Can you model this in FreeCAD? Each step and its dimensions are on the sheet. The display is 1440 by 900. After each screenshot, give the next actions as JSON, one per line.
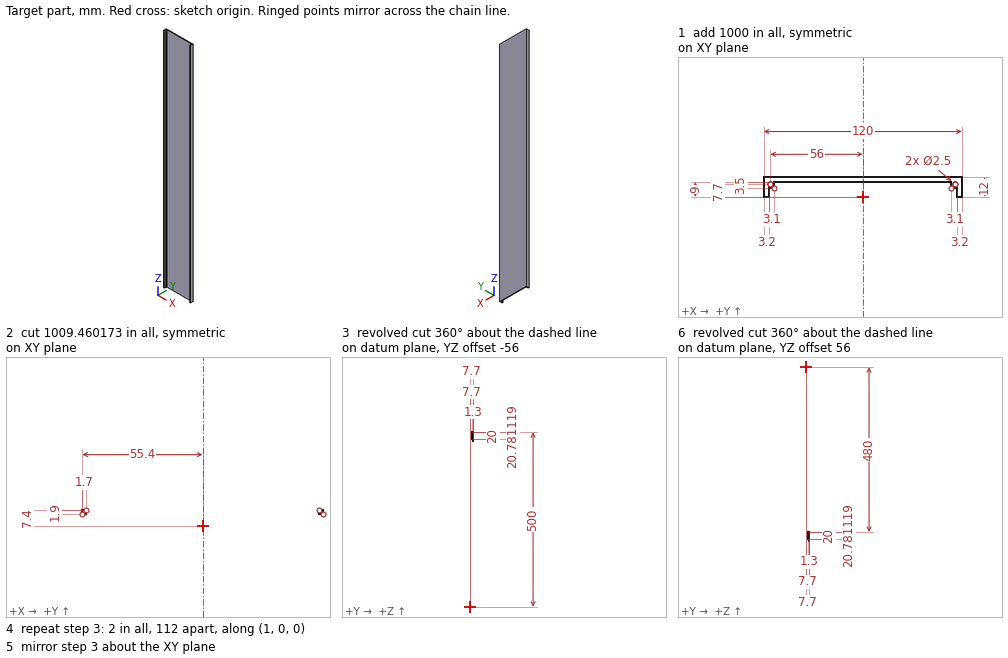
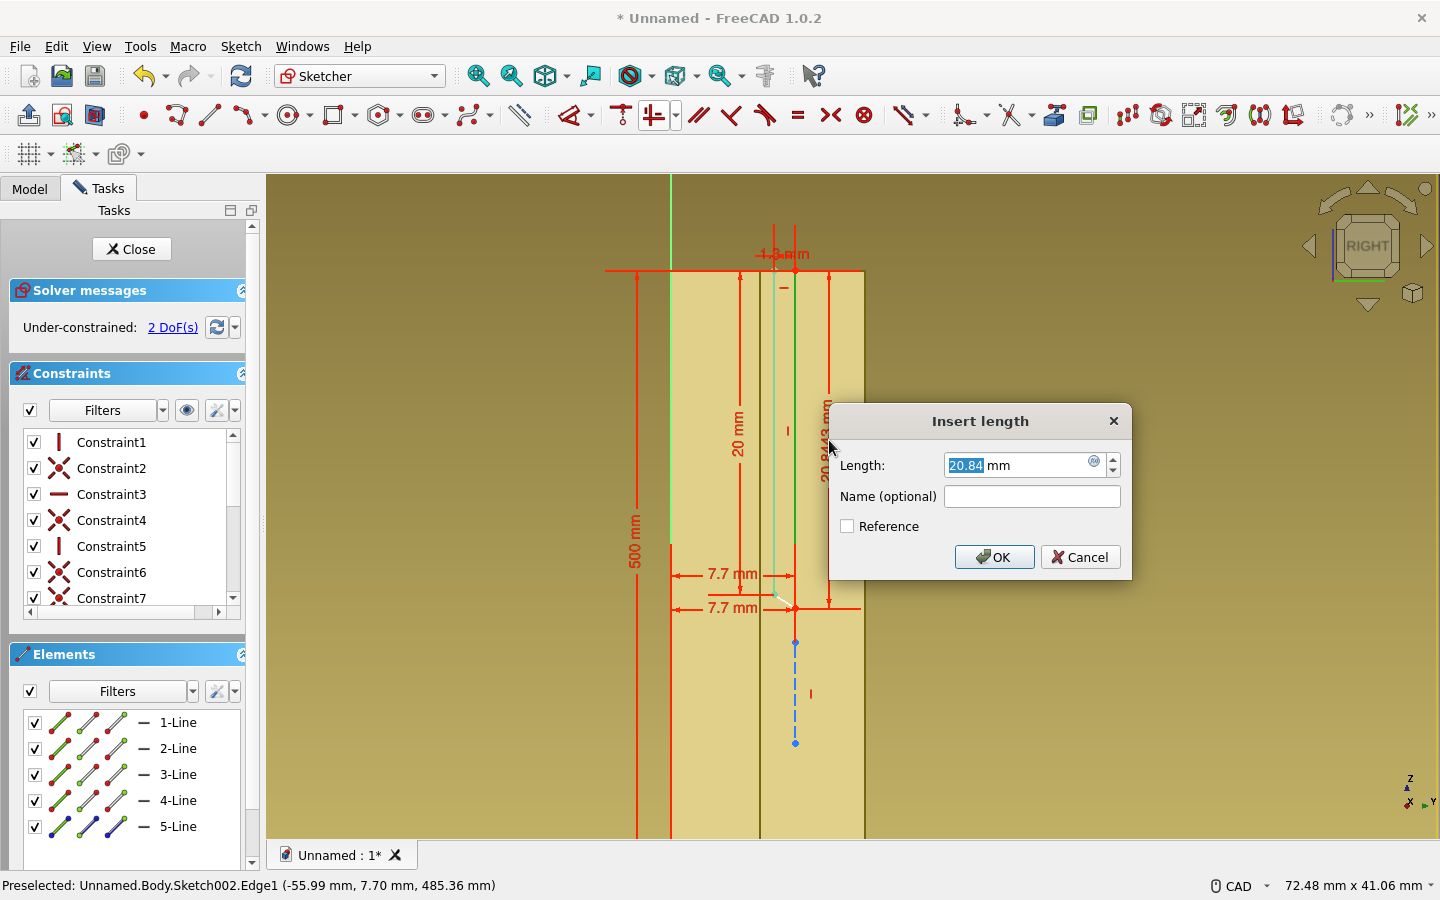
{"action": "type", "text": "20.781119"}
{"action": "key", "text": "Return"}
{"action": "key", "text": "Escape"}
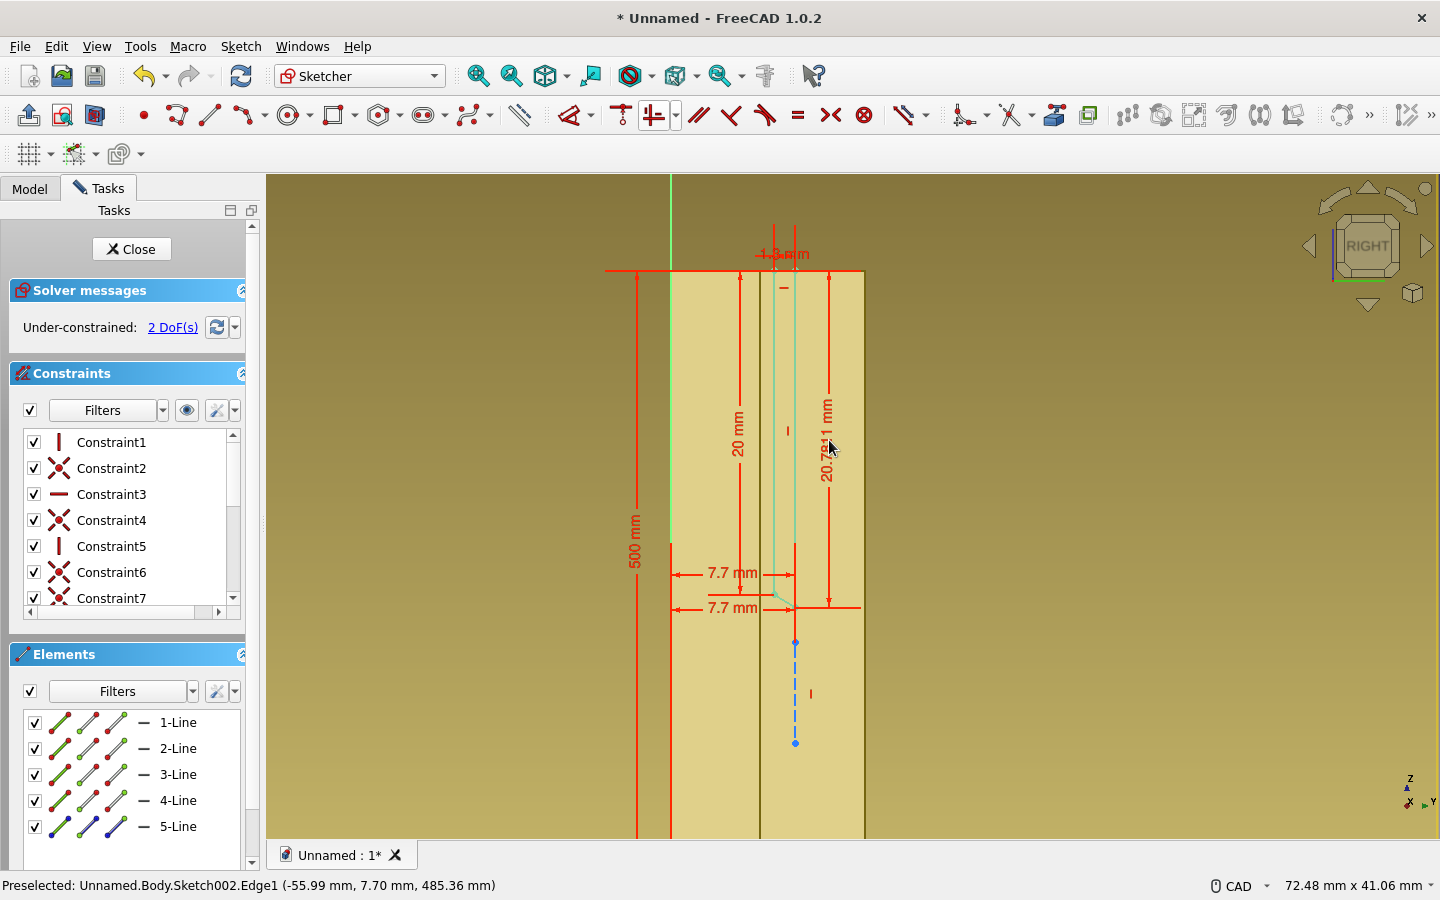
{"action": "left_click", "coordinate": [132, 249]}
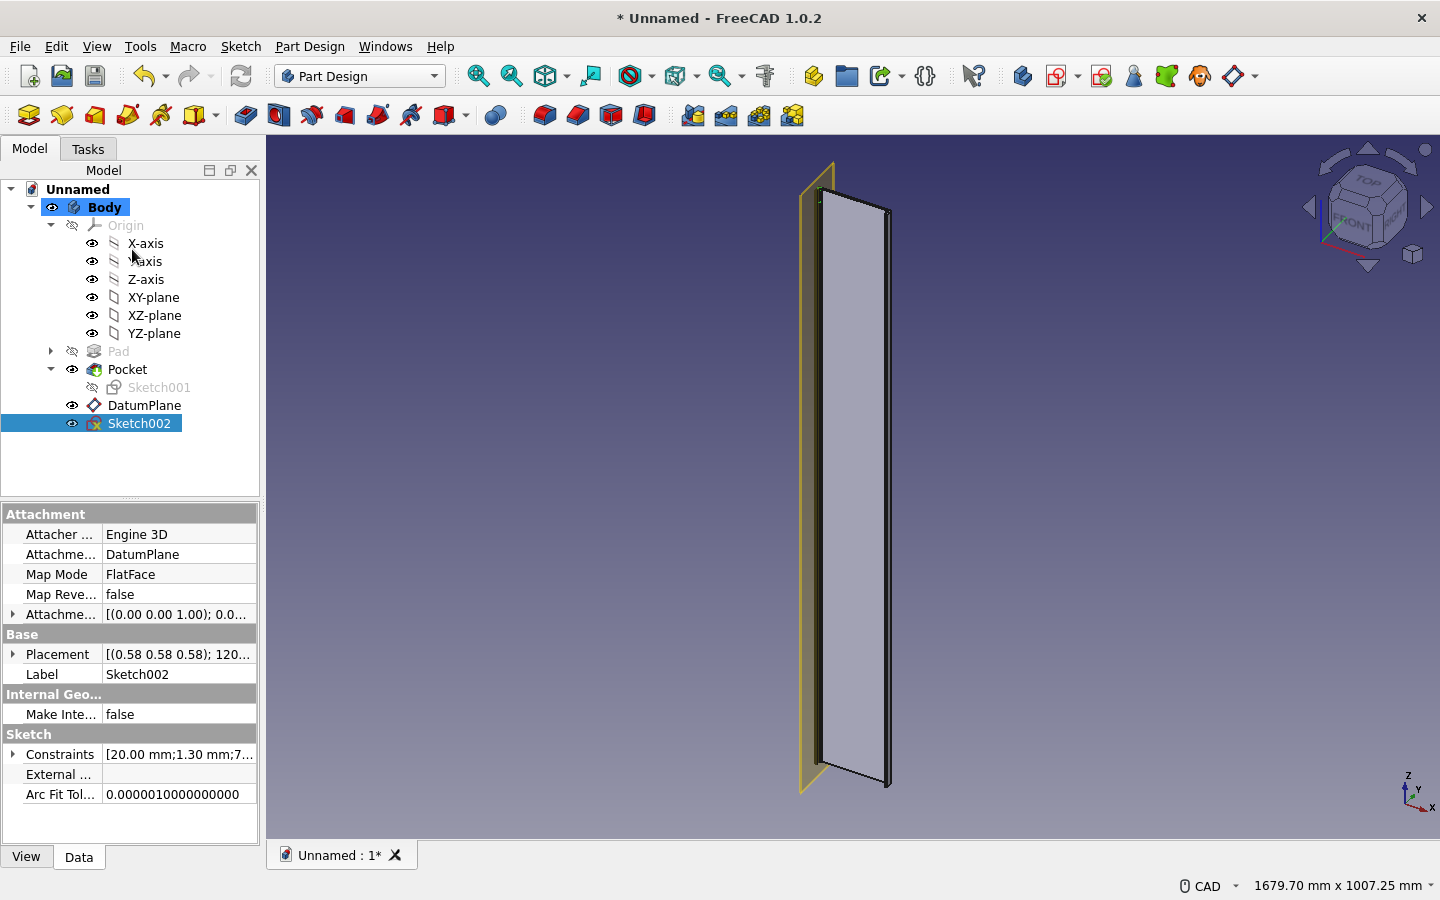
{"action": "left_click", "coordinate": [312, 116]}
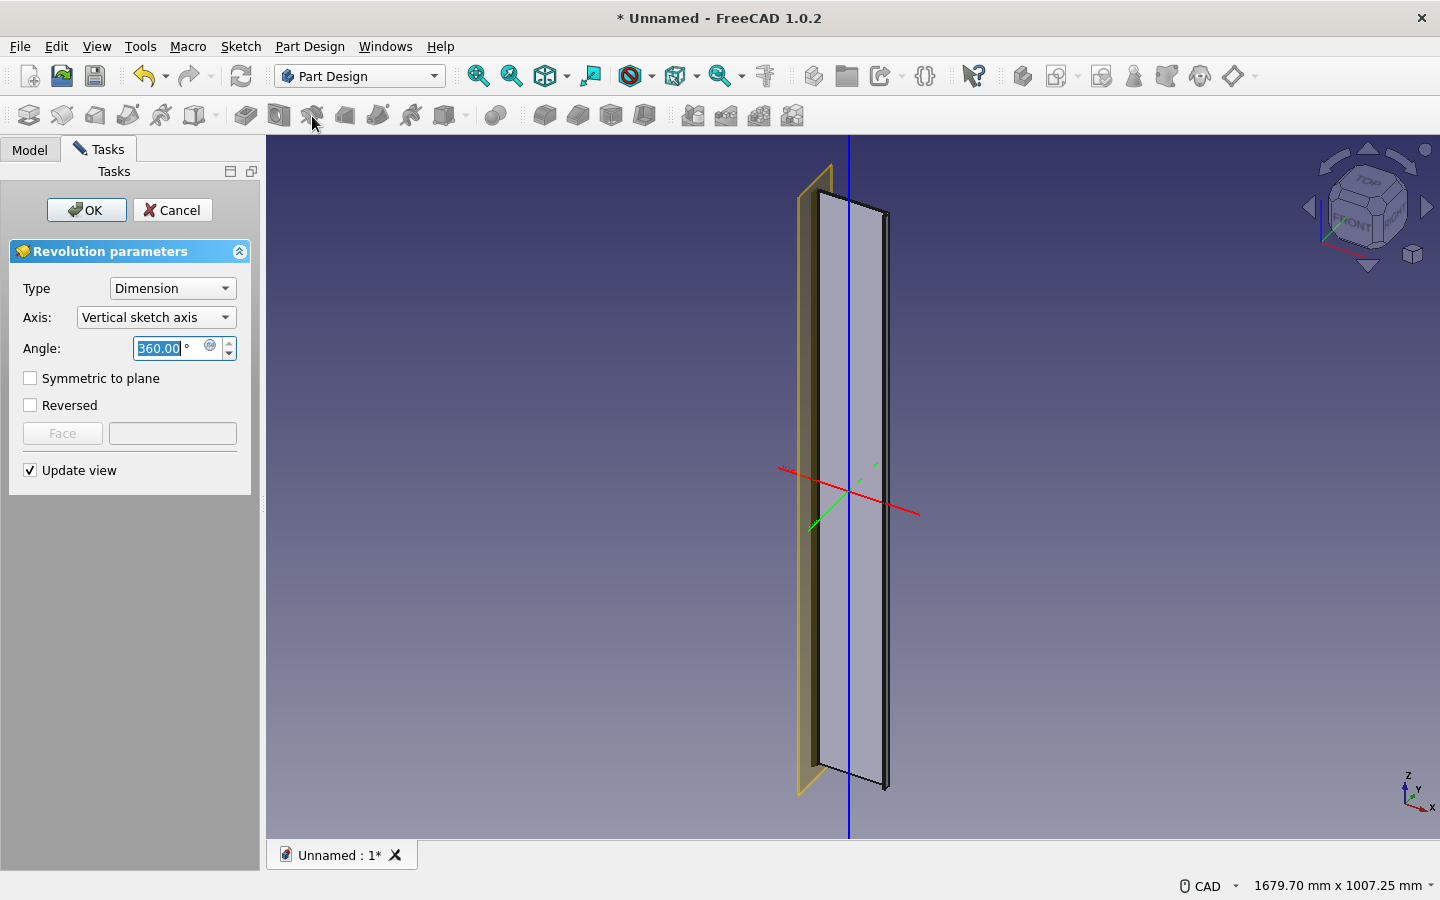
{"action": "left_click", "coordinate": [157, 318]}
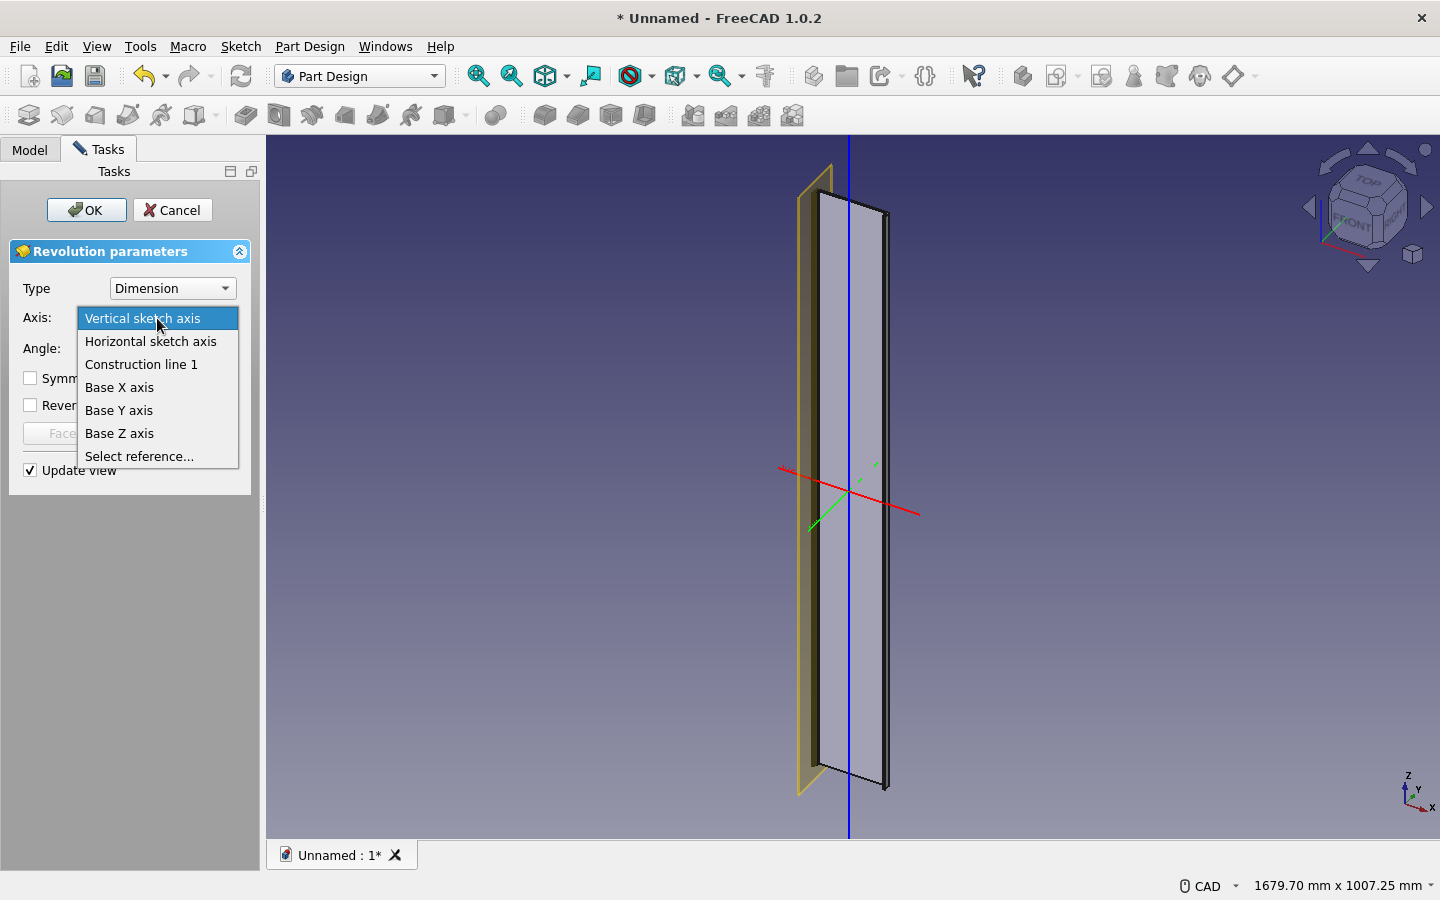
{"action": "left_click", "coordinate": [156, 364]}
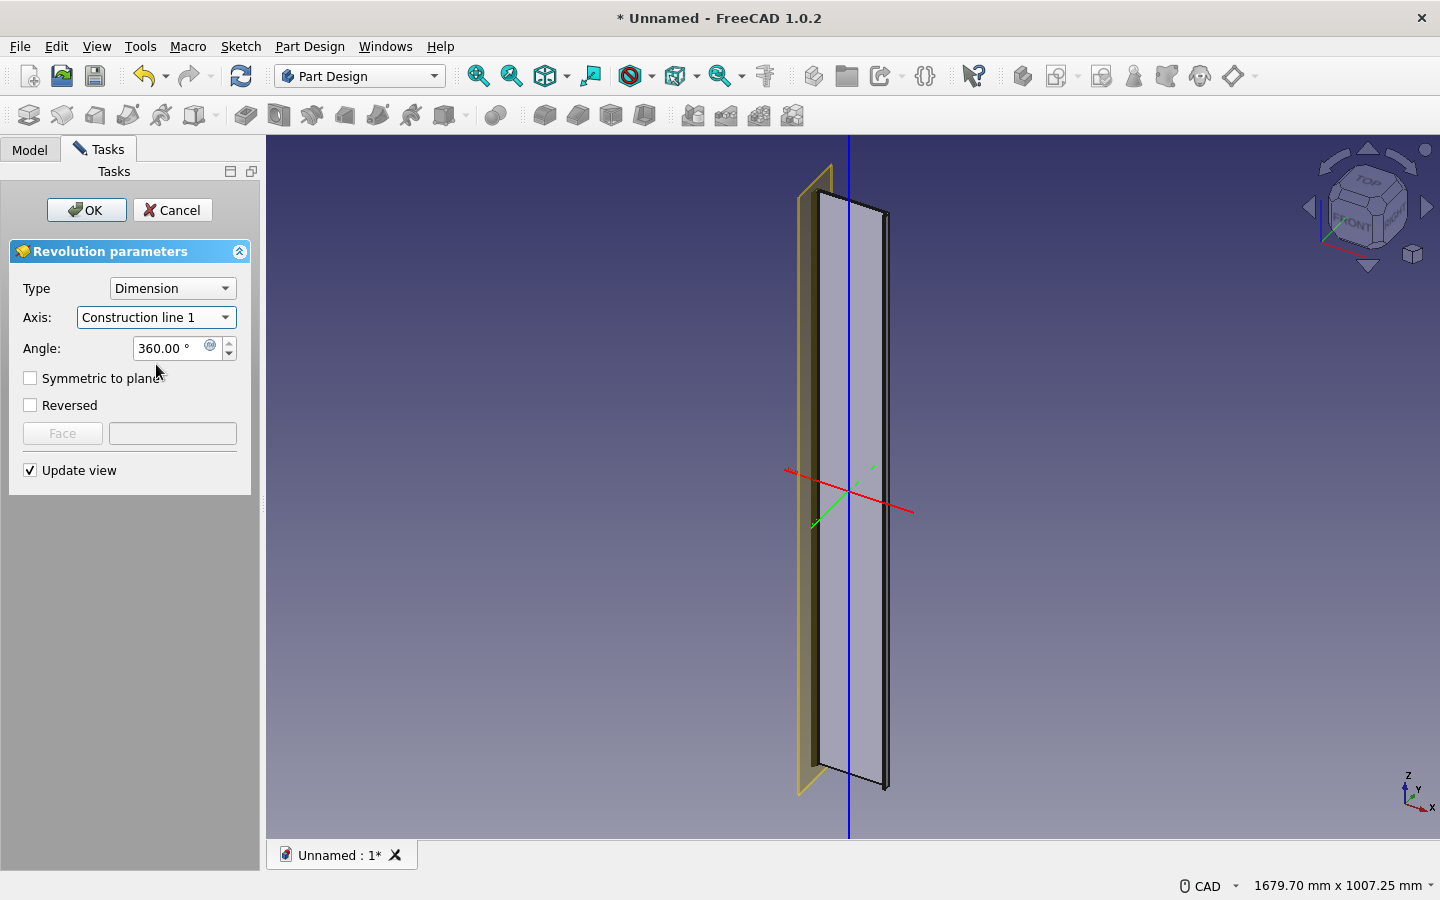
{"action": "left_click", "coordinate": [87, 210]}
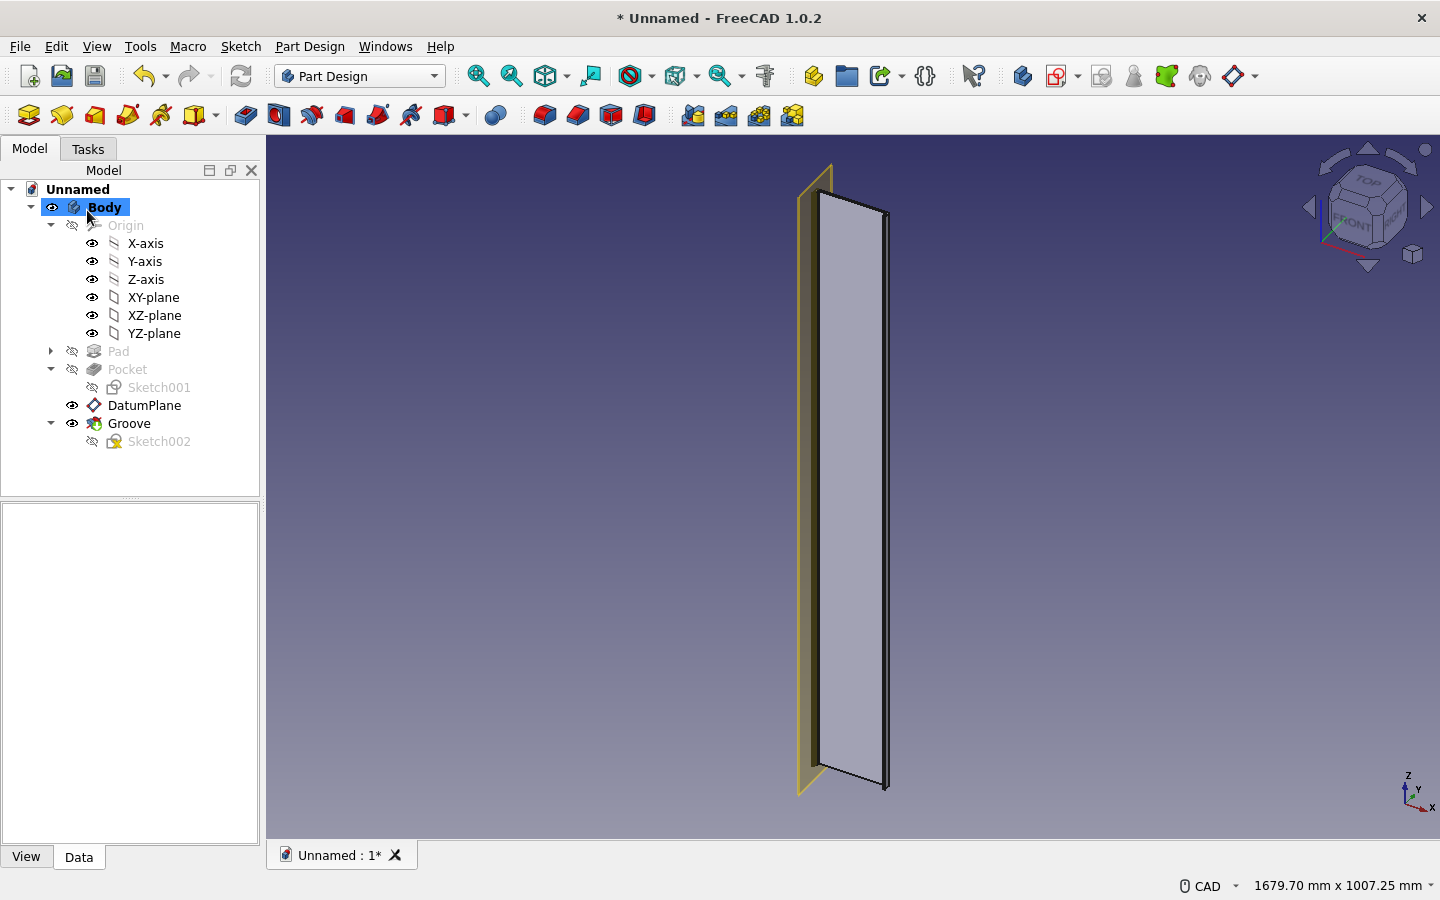
{"action": "left_click", "coordinate": [117, 405]}
{"action": "key", "text": "space"}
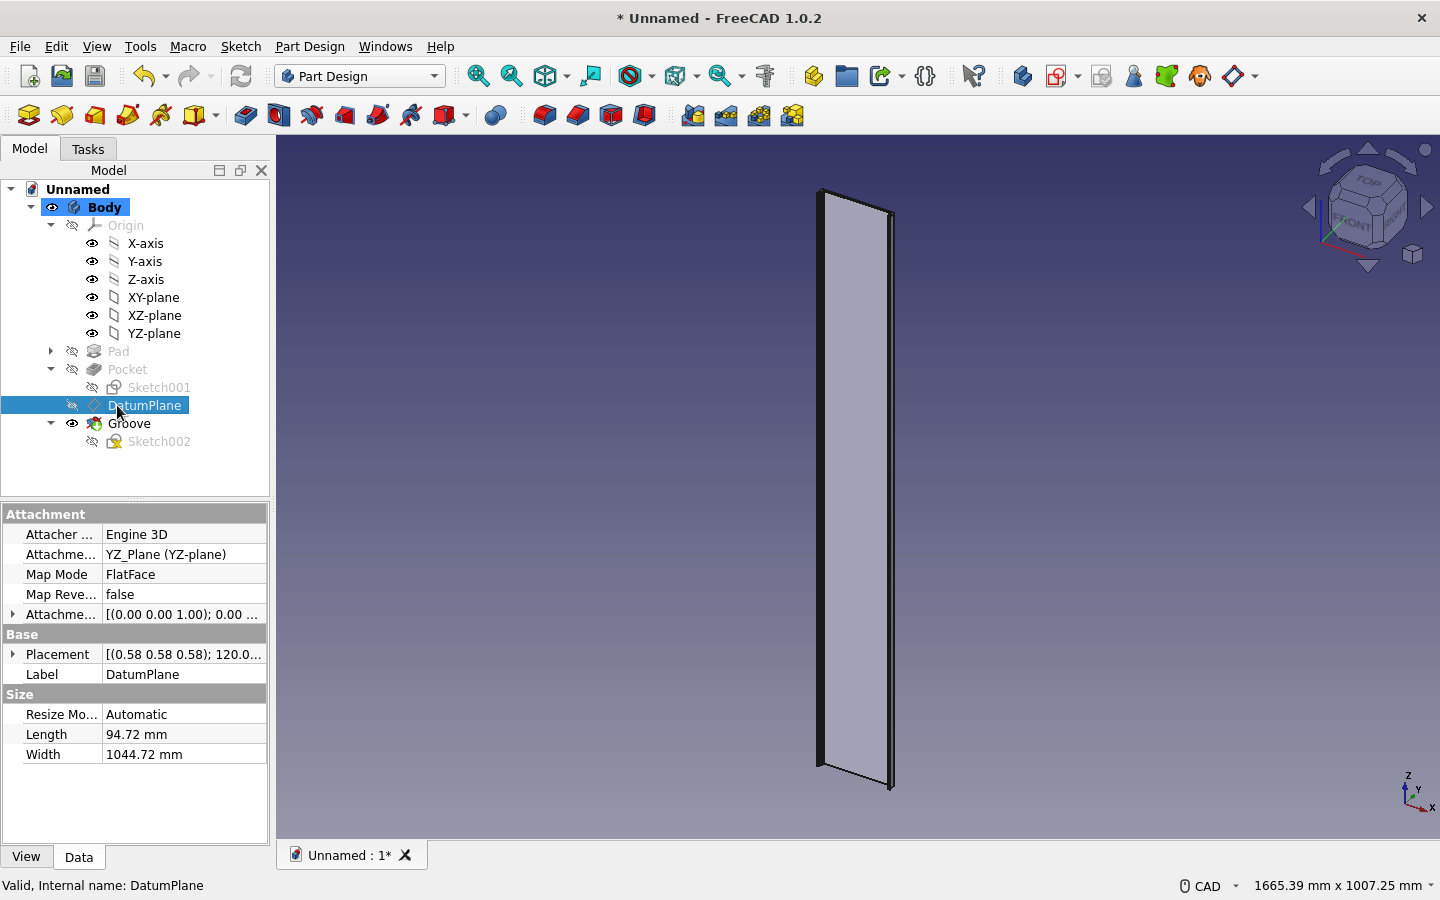
{"action": "left_click", "coordinate": [117, 423]}